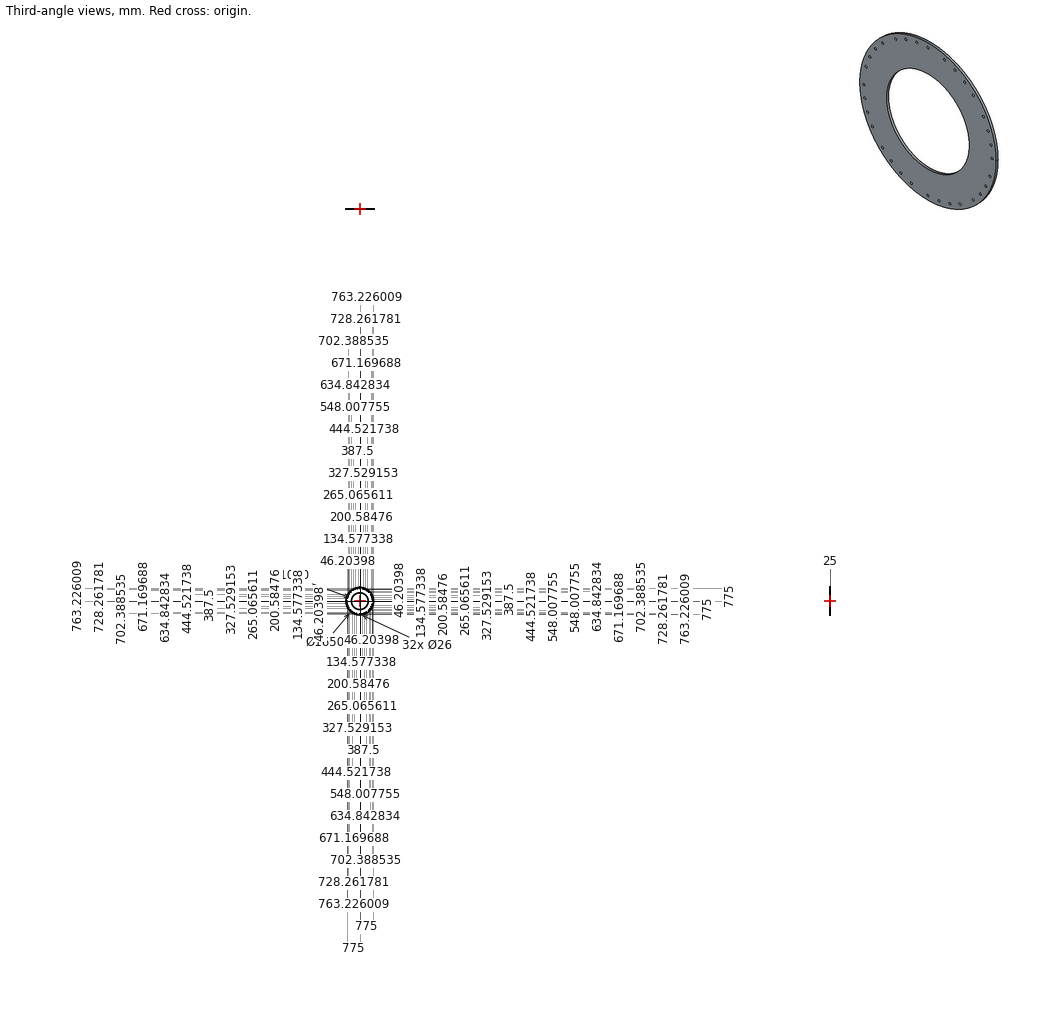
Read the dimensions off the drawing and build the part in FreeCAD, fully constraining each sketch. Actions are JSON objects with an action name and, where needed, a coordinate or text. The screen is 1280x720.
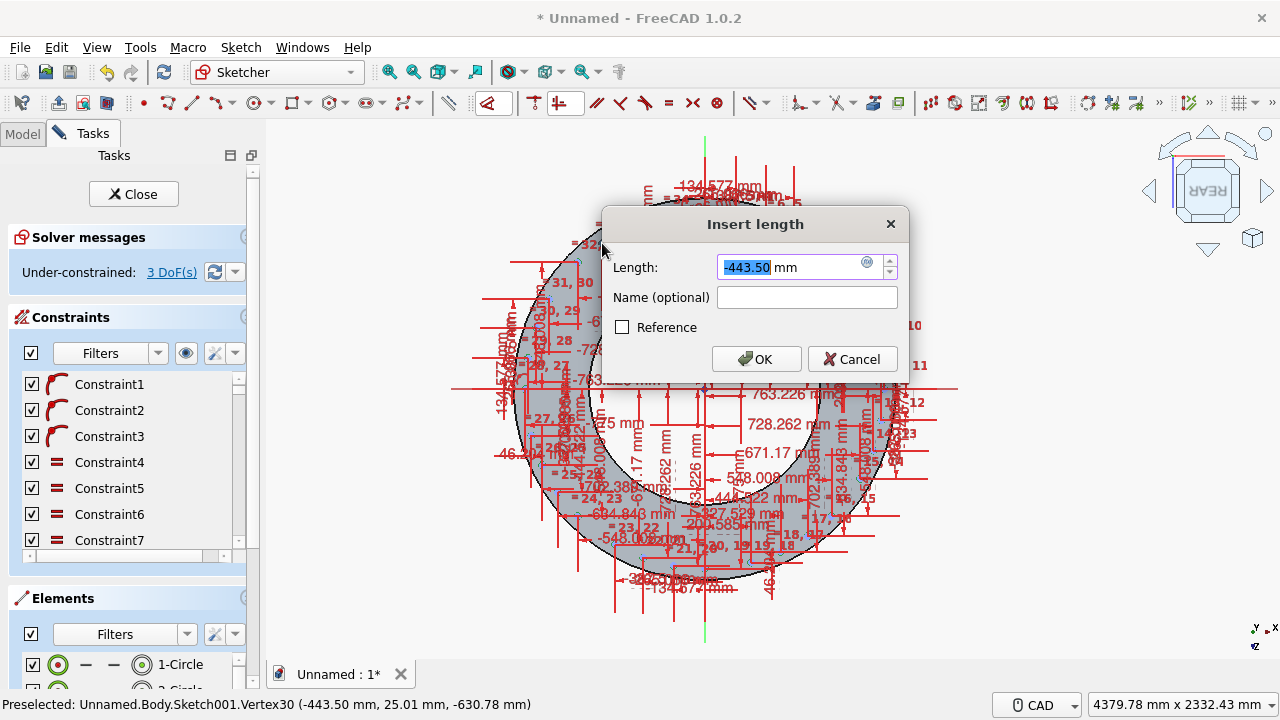
{"action": "type", "text": "-444.521738"}
{"action": "key", "text": "Return"}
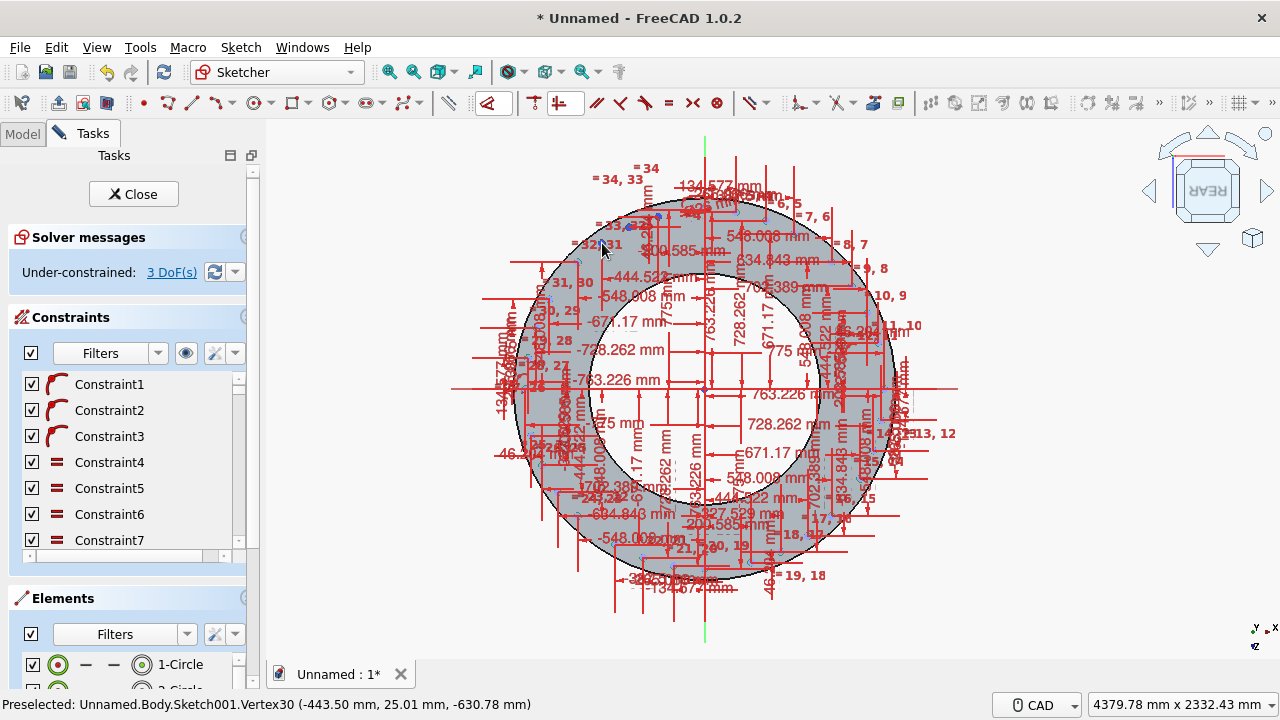
{"action": "left_click", "coordinate": [602, 243]}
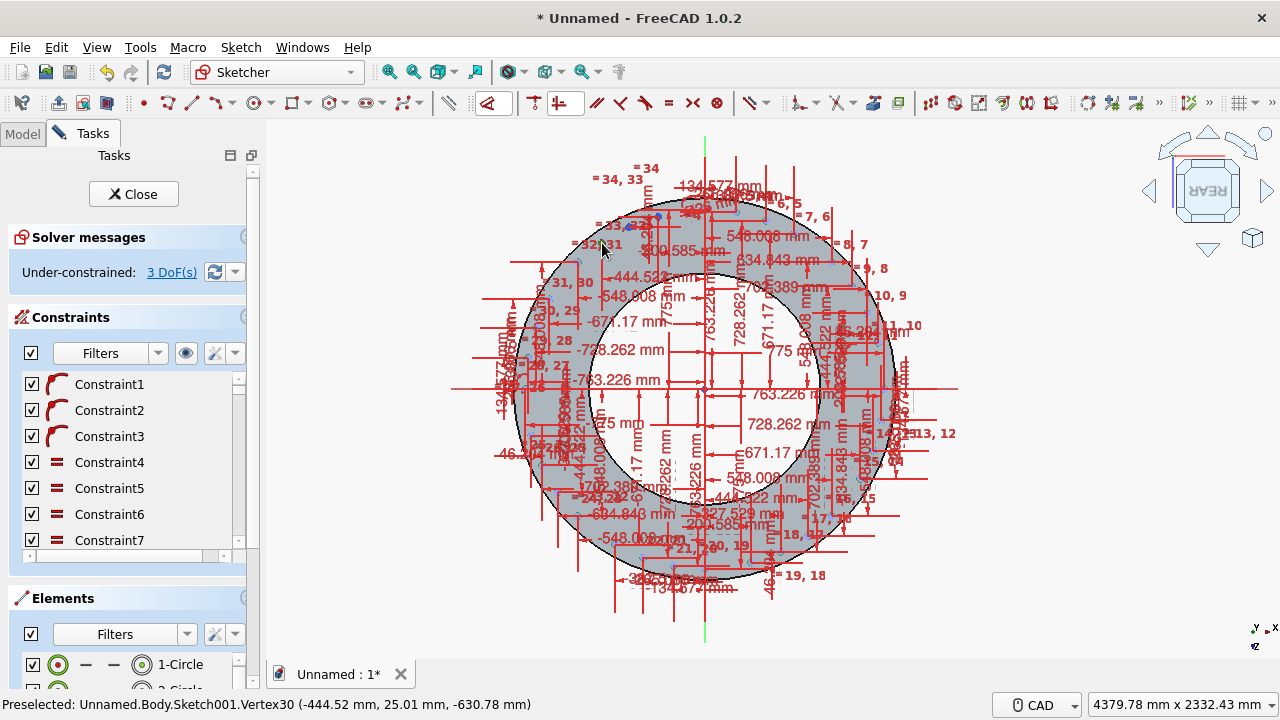
{"action": "key", "text": "i"}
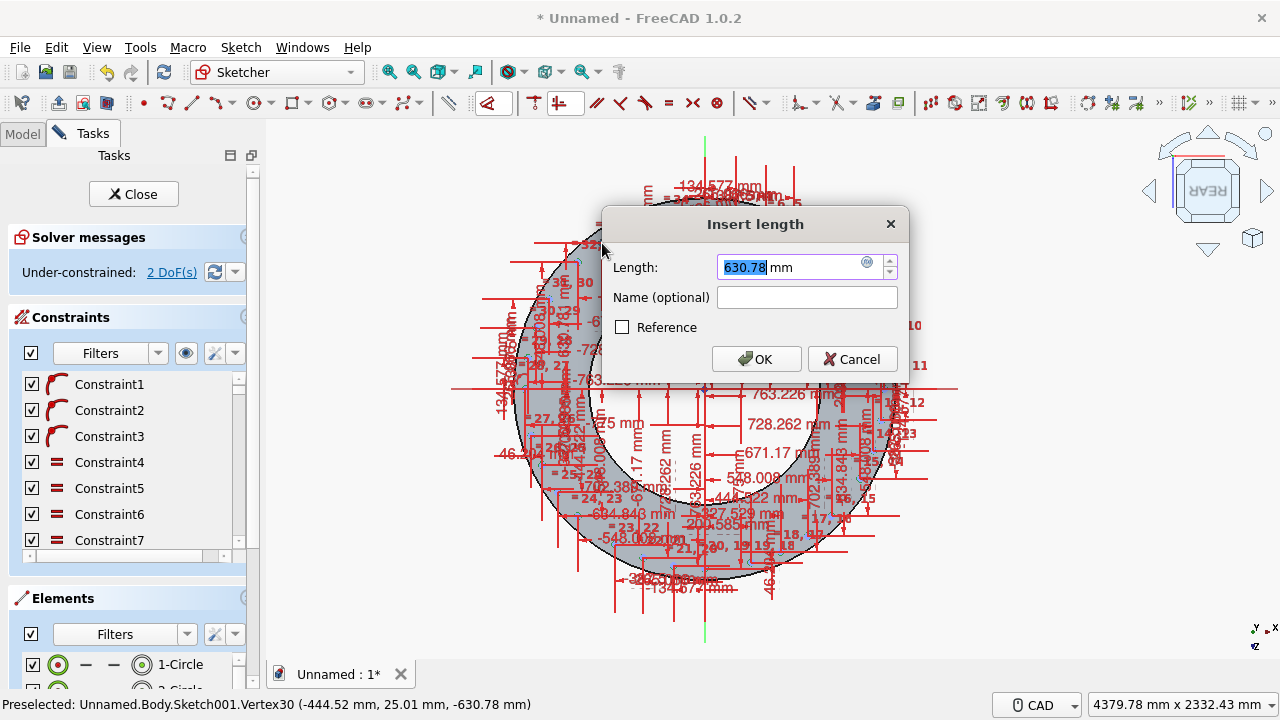
{"action": "type", "text": "634.842834"}
{"action": "key", "text": "Return"}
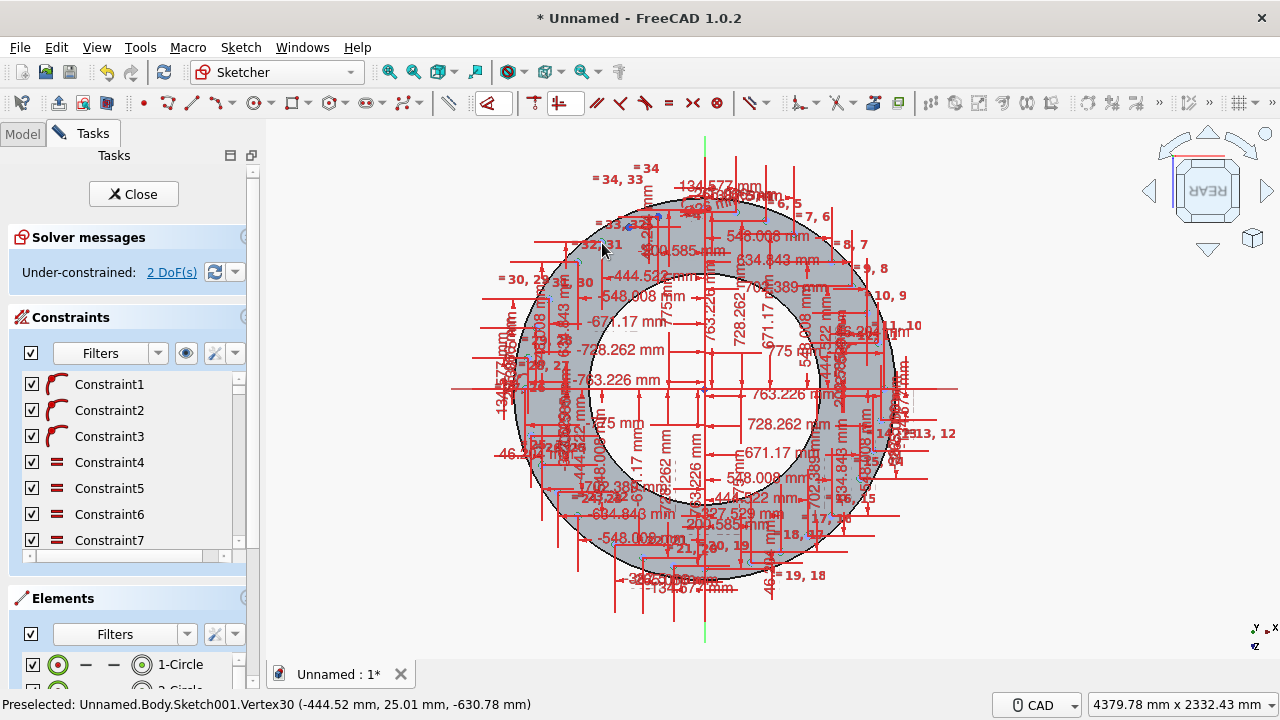
{"action": "left_click", "coordinate": [629, 227]}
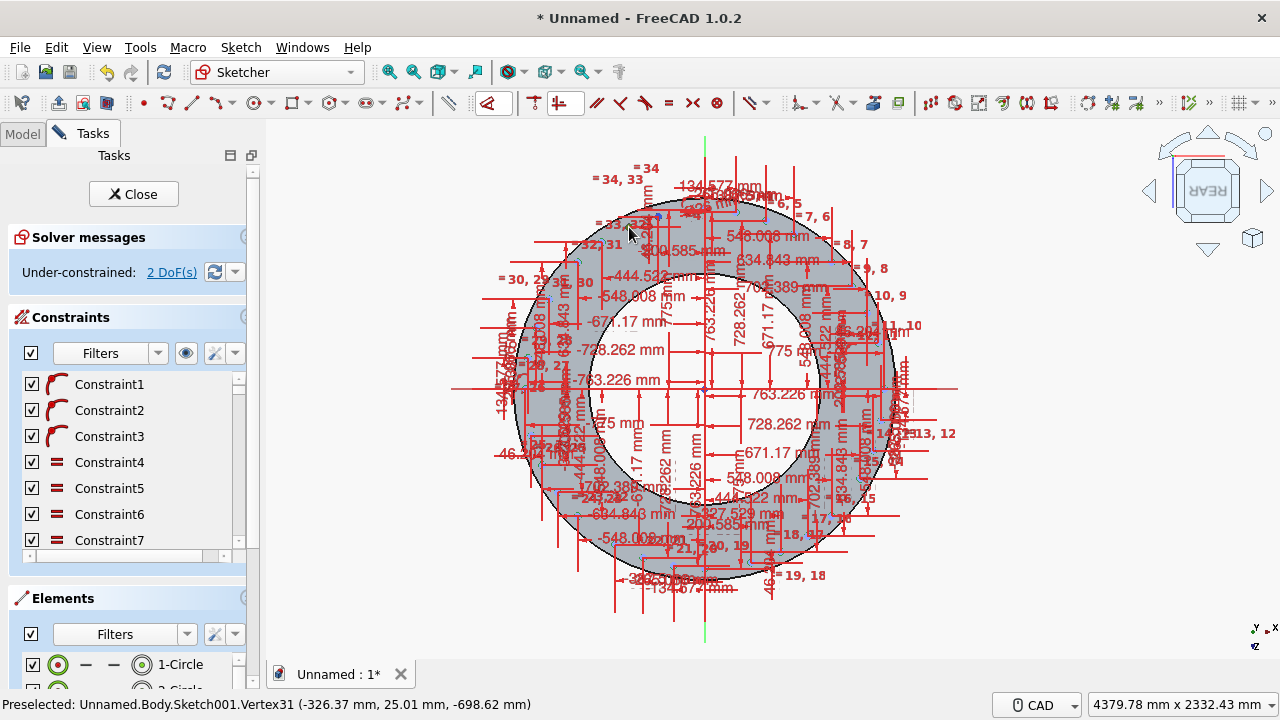
{"action": "key", "text": "l"}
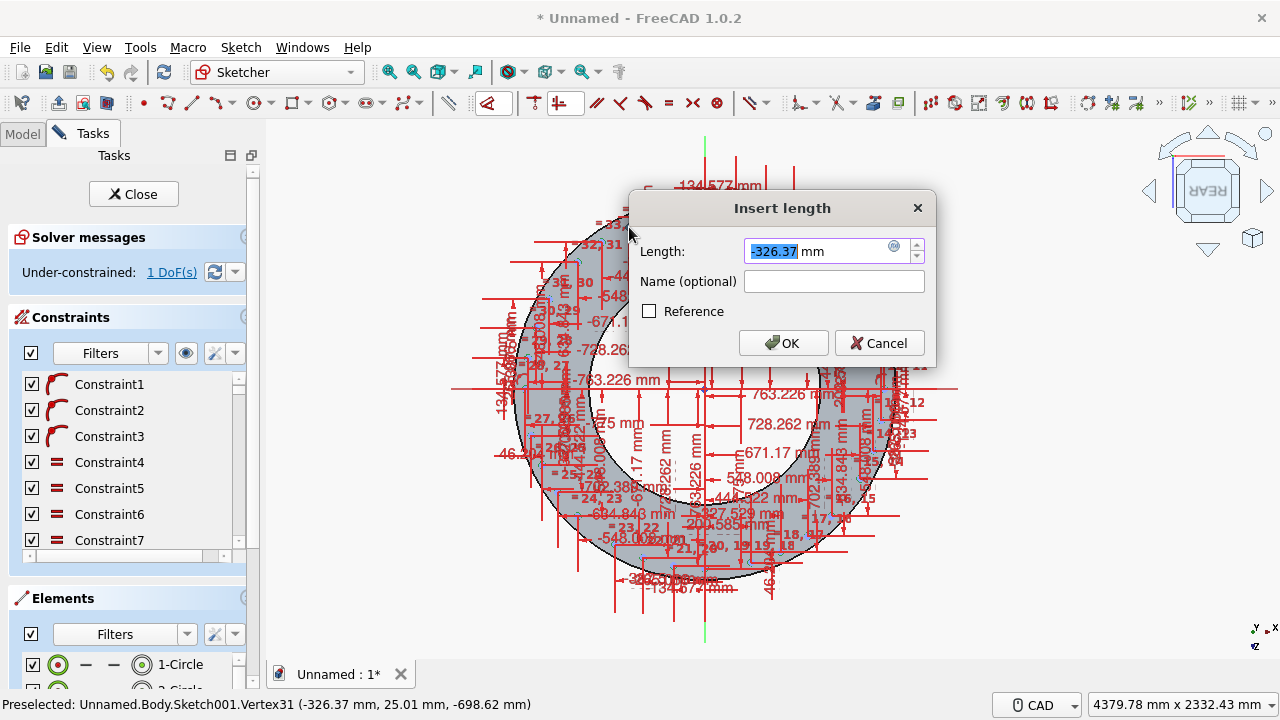
{"action": "type", "text": "-327.529153"}
{"action": "key", "text": "Return"}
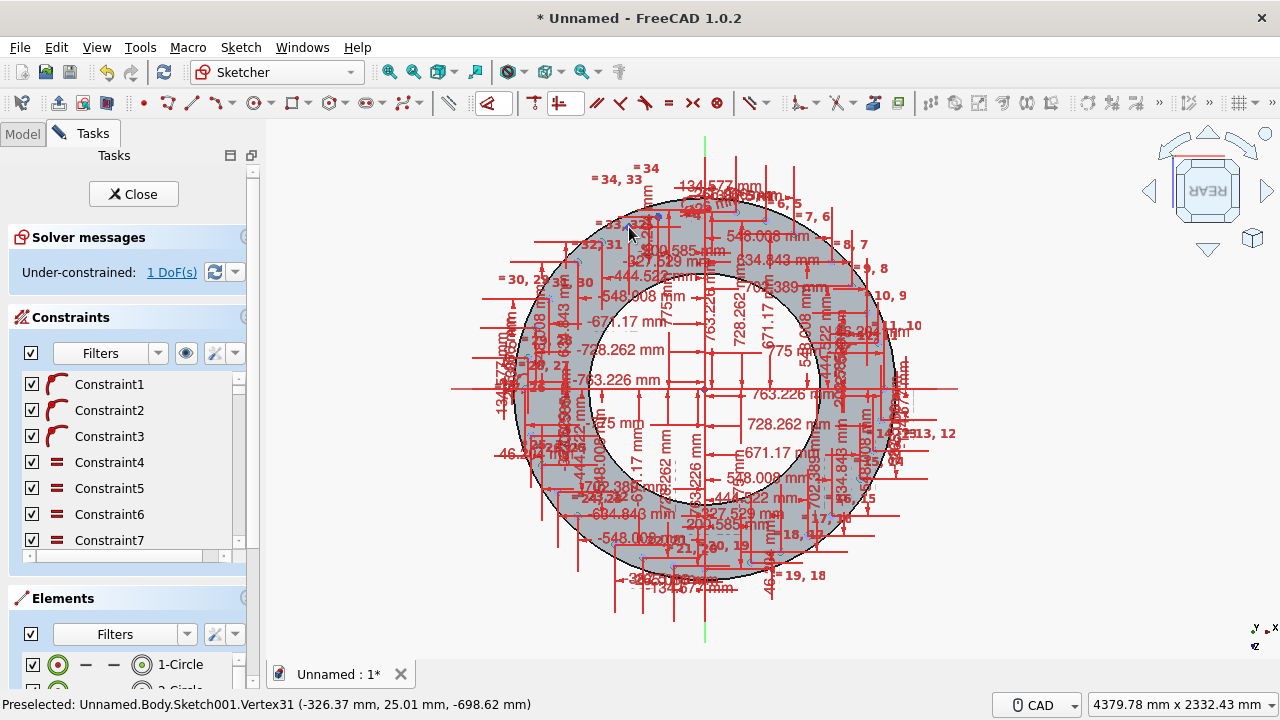
{"action": "left_click", "coordinate": [629, 227]}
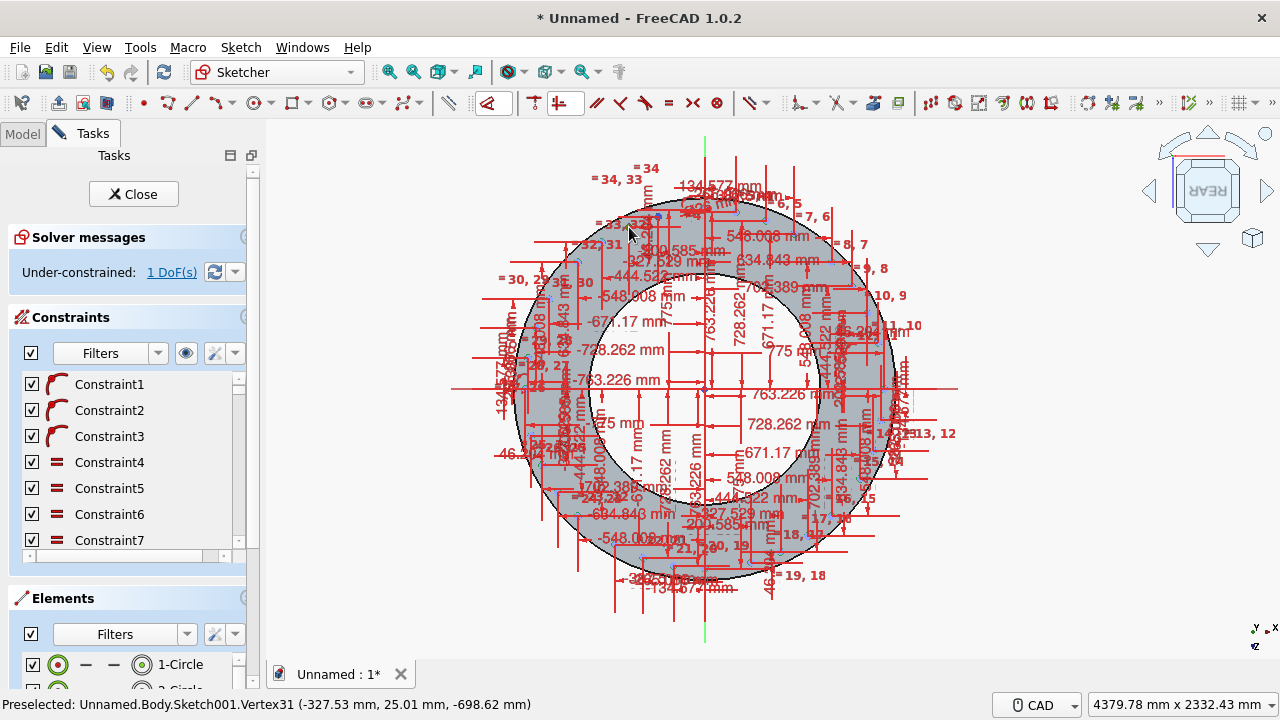
{"action": "left_click", "coordinate": [506, 104]}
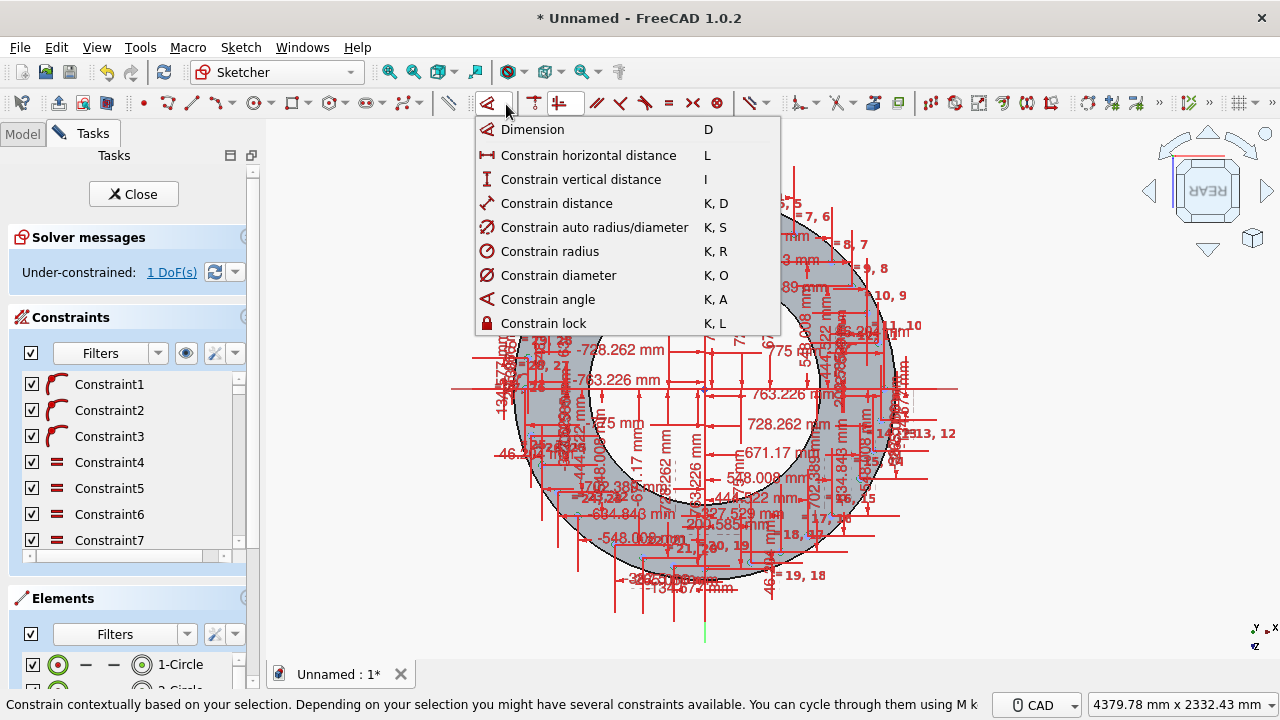
{"action": "left_click", "coordinate": [628, 179]}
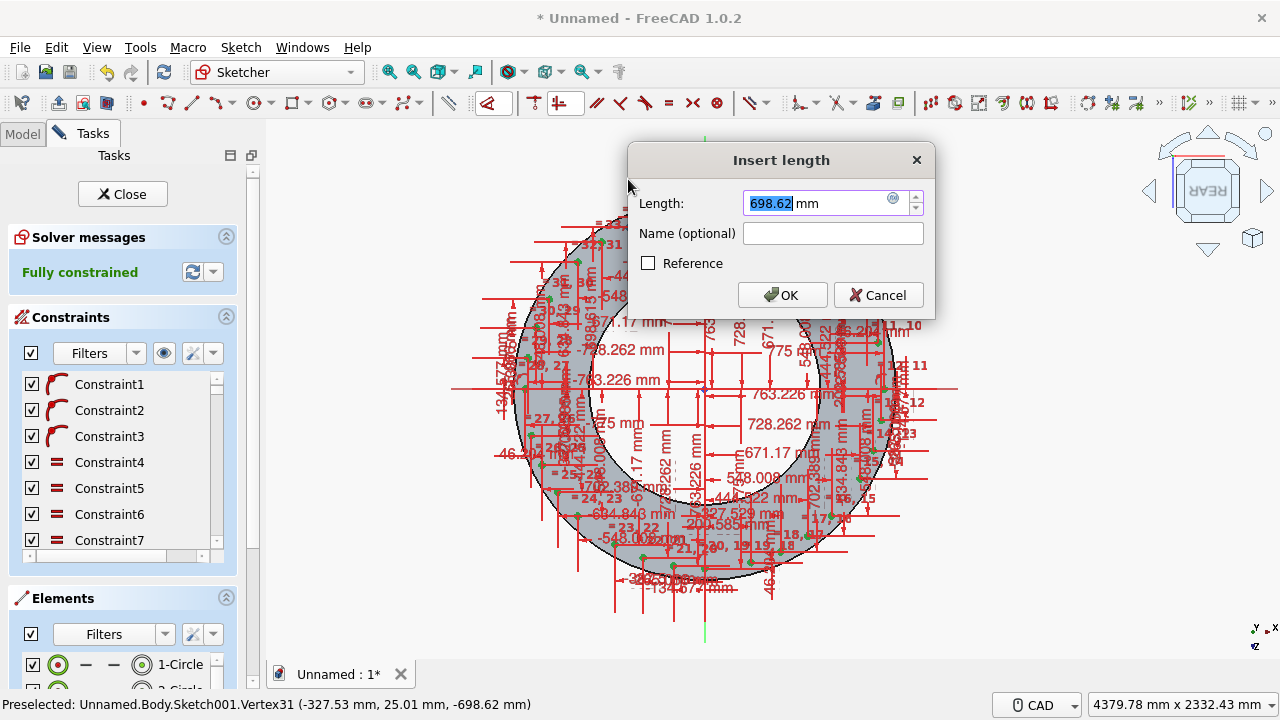
{"action": "type", "text": "702.388535"}
{"action": "key", "text": "Return"}